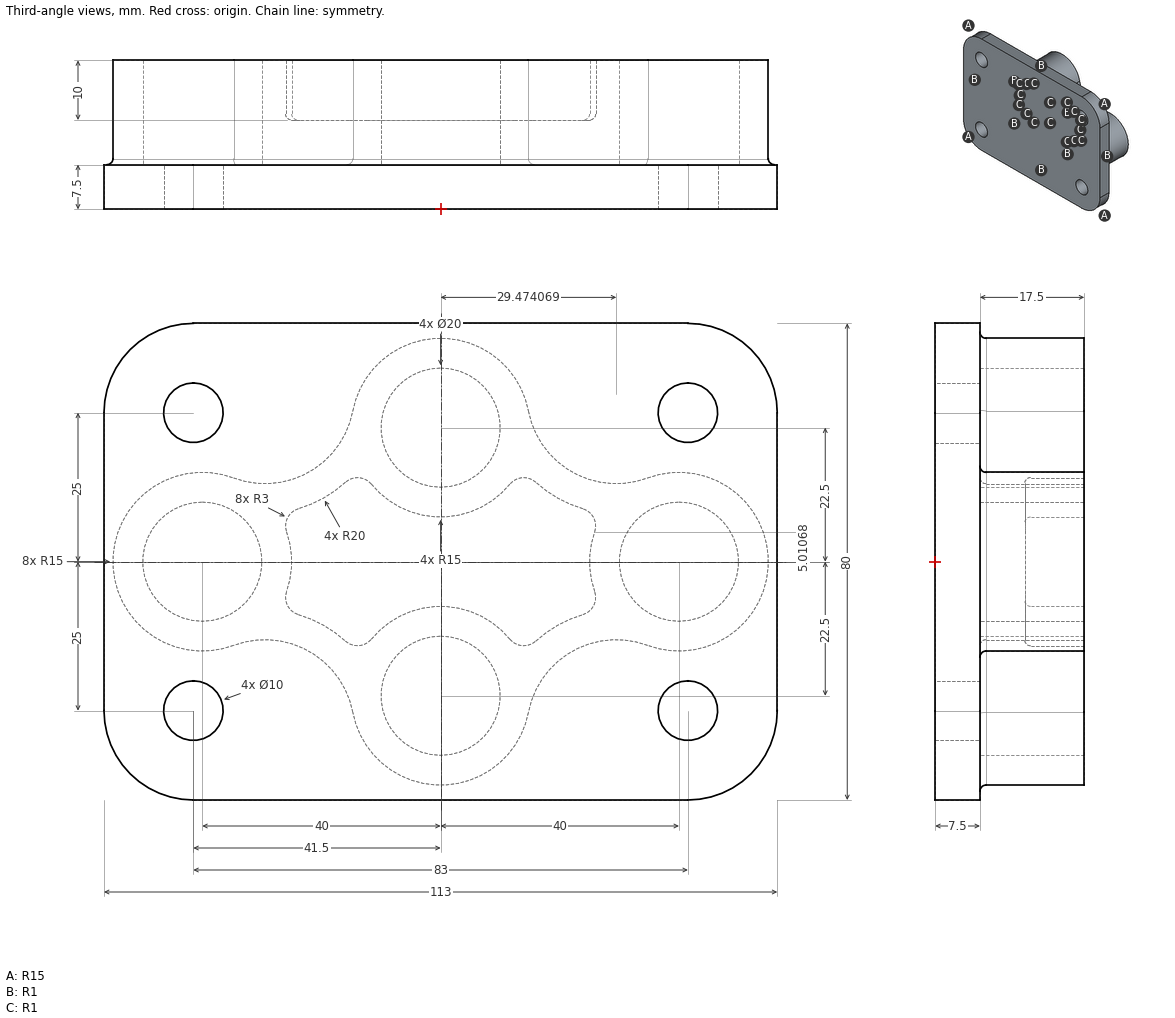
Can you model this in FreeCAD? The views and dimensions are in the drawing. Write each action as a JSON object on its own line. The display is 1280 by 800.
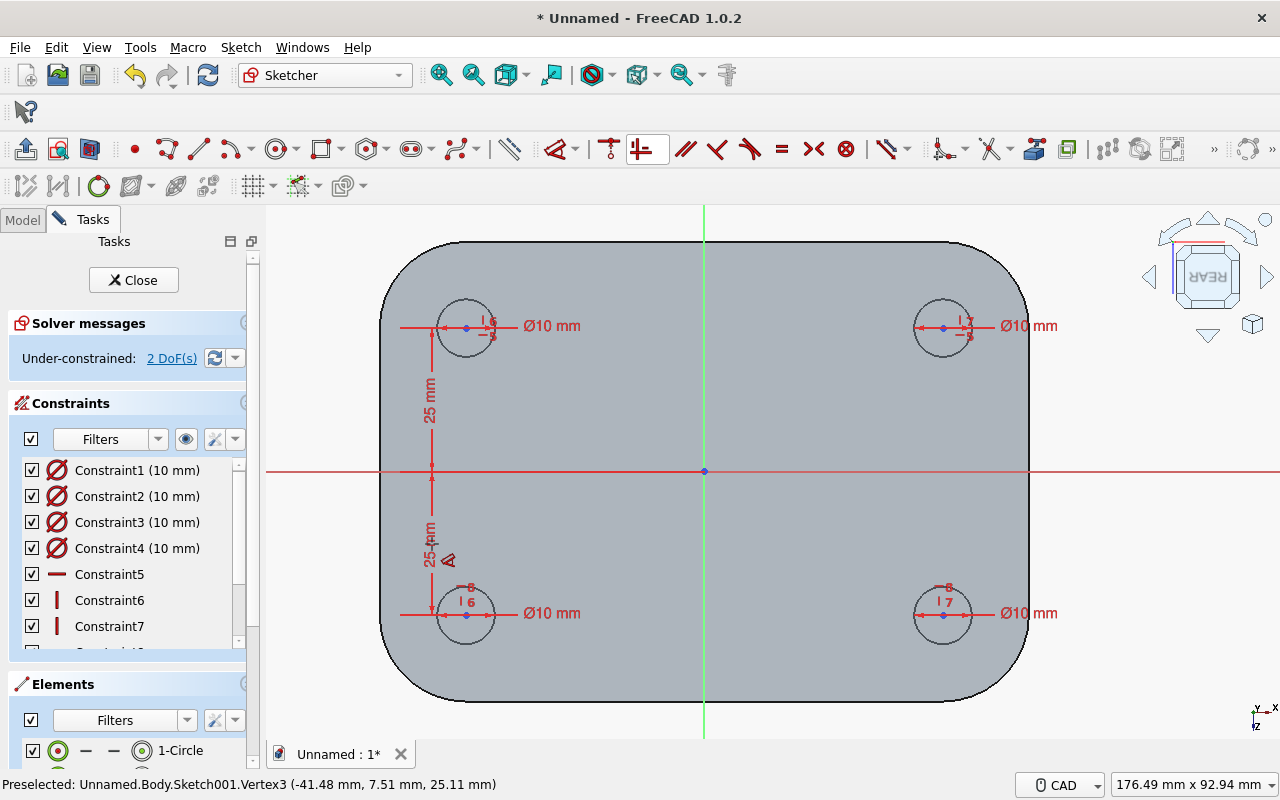
{"action": "left_click", "coordinate": [466, 328]}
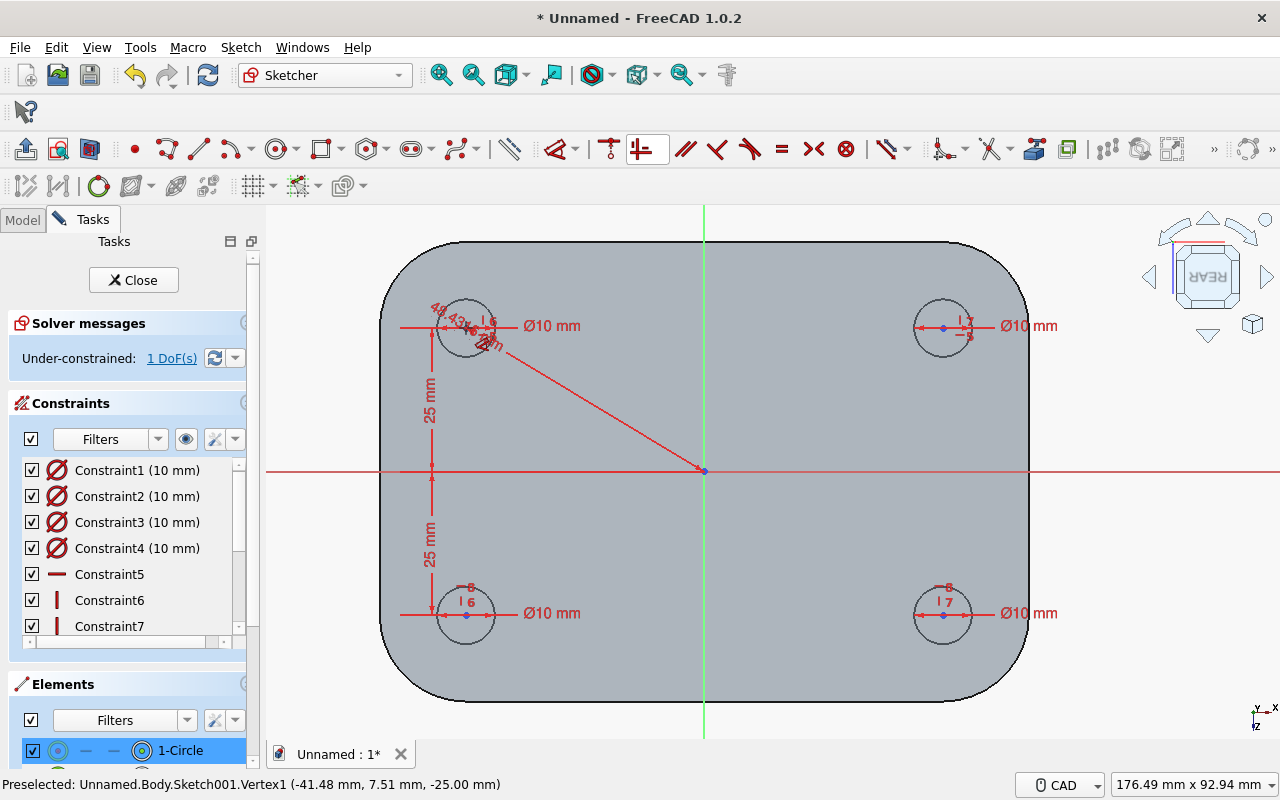
{"action": "left_click", "coordinate": [943, 328]}
{"action": "left_click", "coordinate": [595, 294]}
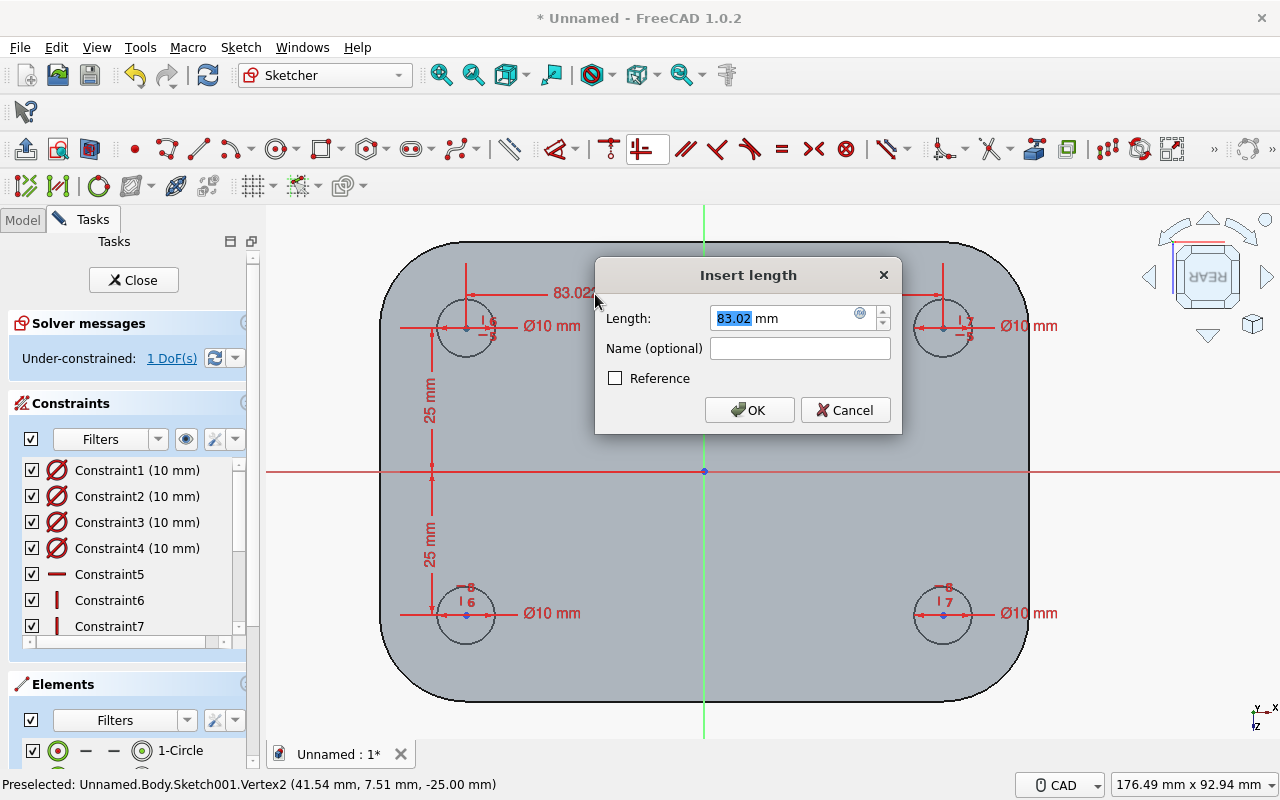
{"action": "type", "text": "83"}
{"action": "key", "text": "Return"}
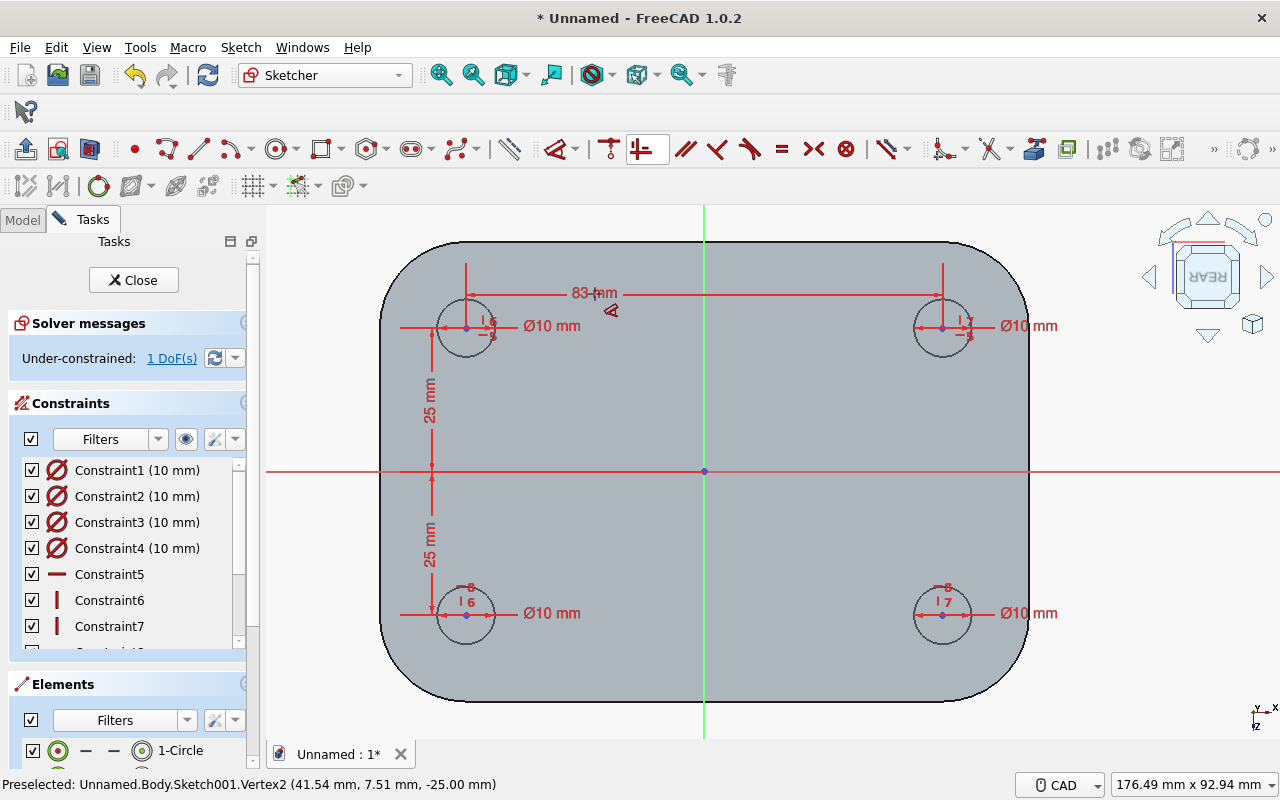
{"action": "left_click", "coordinate": [466, 328]}
{"action": "left_click", "coordinate": [502, 294]}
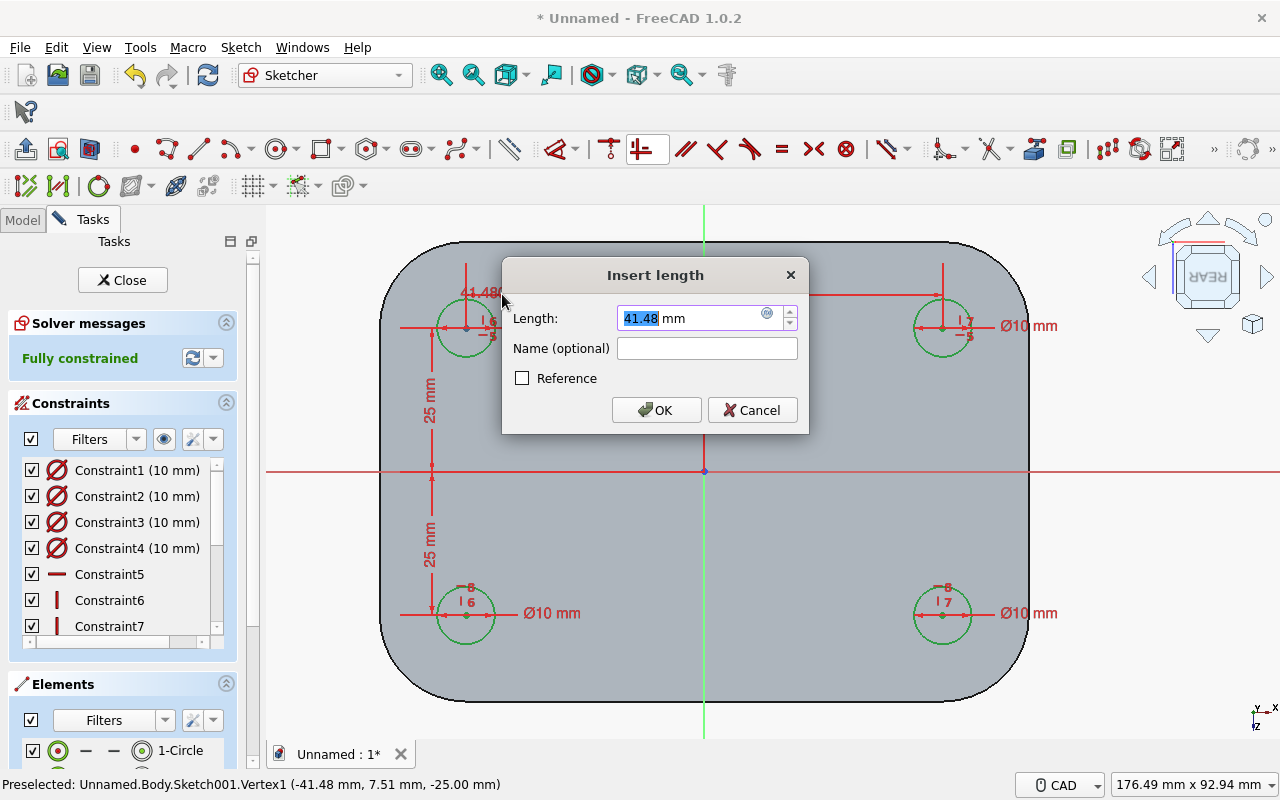
{"action": "type", "text": "41.5"}
{"action": "key", "text": "Return"}
{"action": "key", "text": "Escape"}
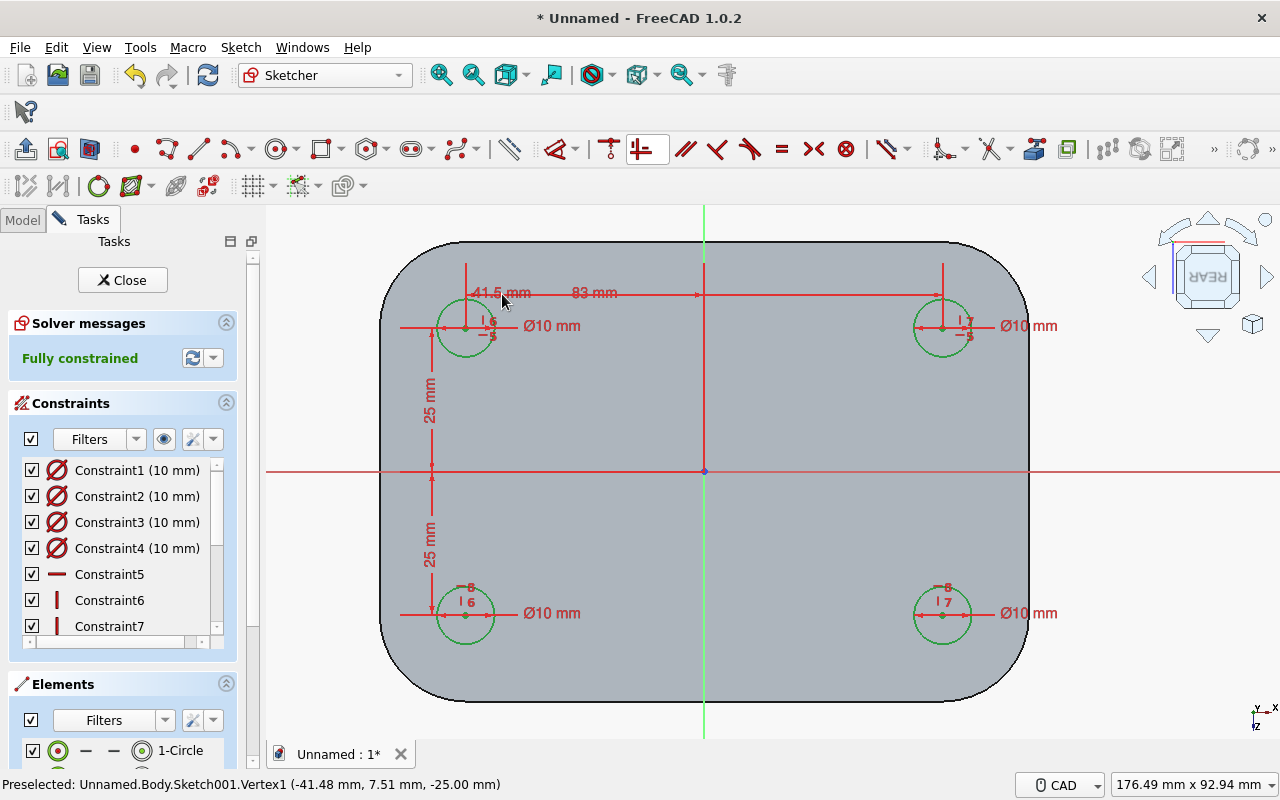
{"action": "left_click", "coordinate": [123, 280]}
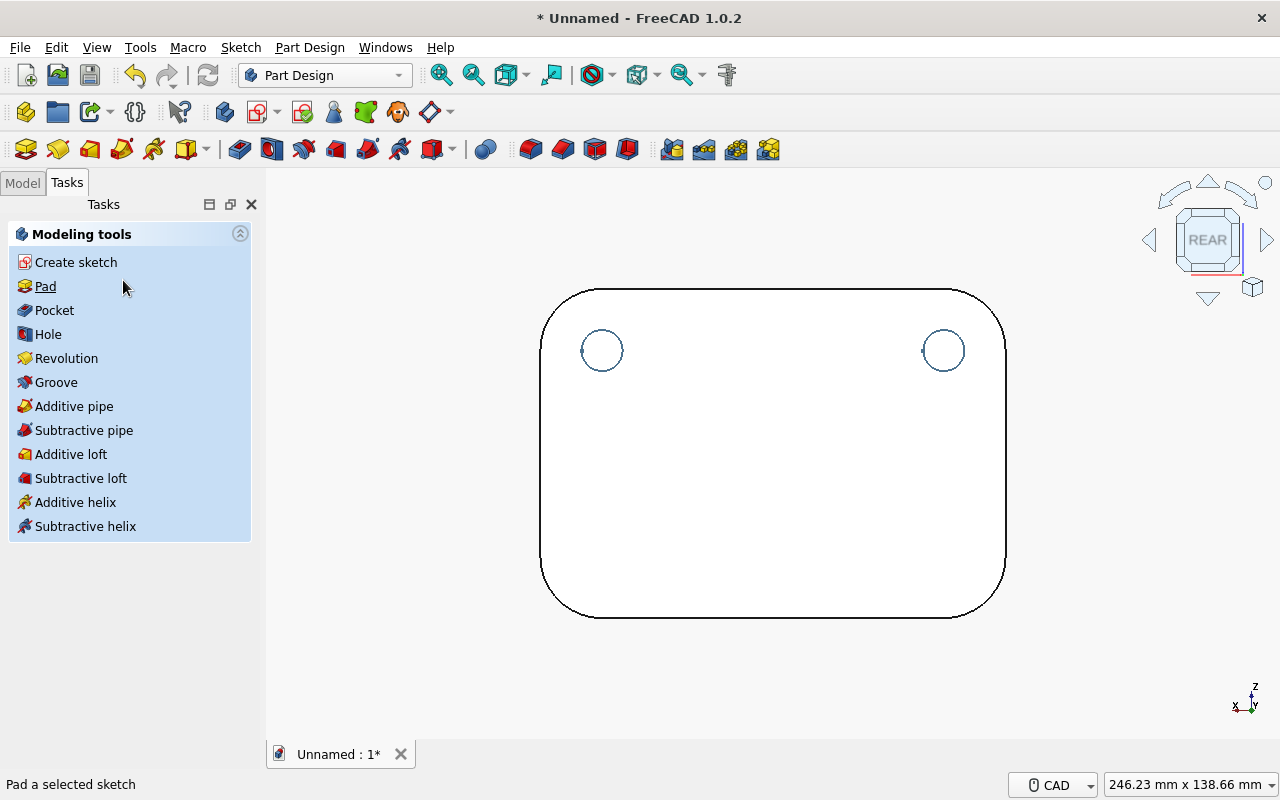
{"action": "left_click", "coordinate": [240, 150]}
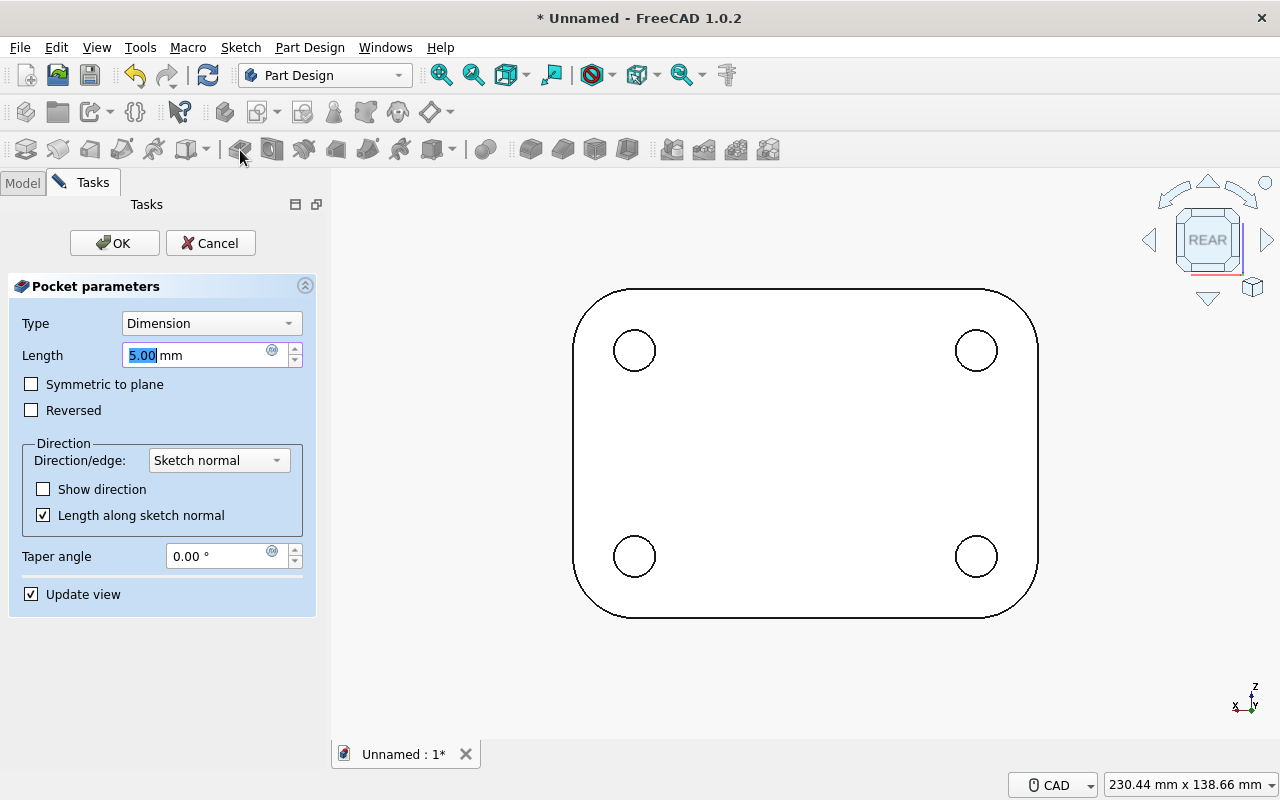
{"action": "type", "text": "7.5"}
{"action": "key", "text": "Tab"}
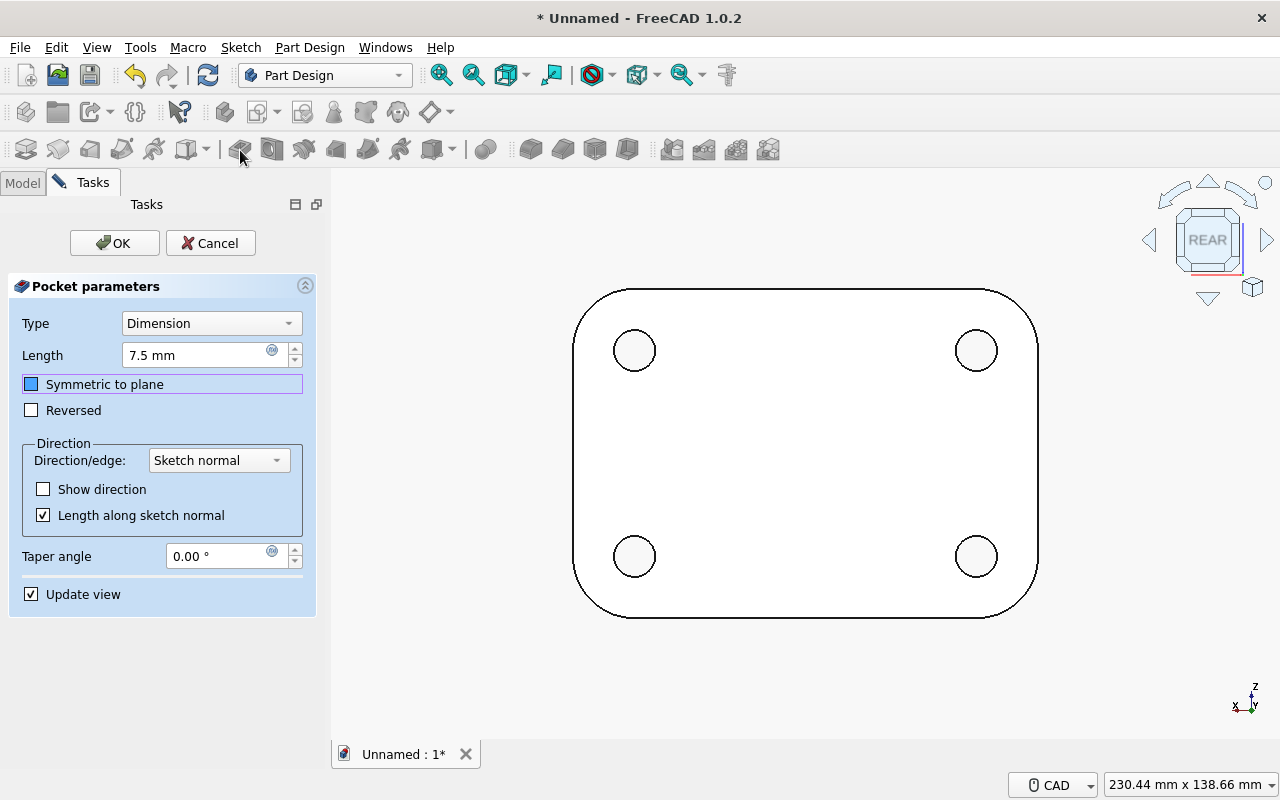
{"action": "left_click", "coordinate": [115, 243]}